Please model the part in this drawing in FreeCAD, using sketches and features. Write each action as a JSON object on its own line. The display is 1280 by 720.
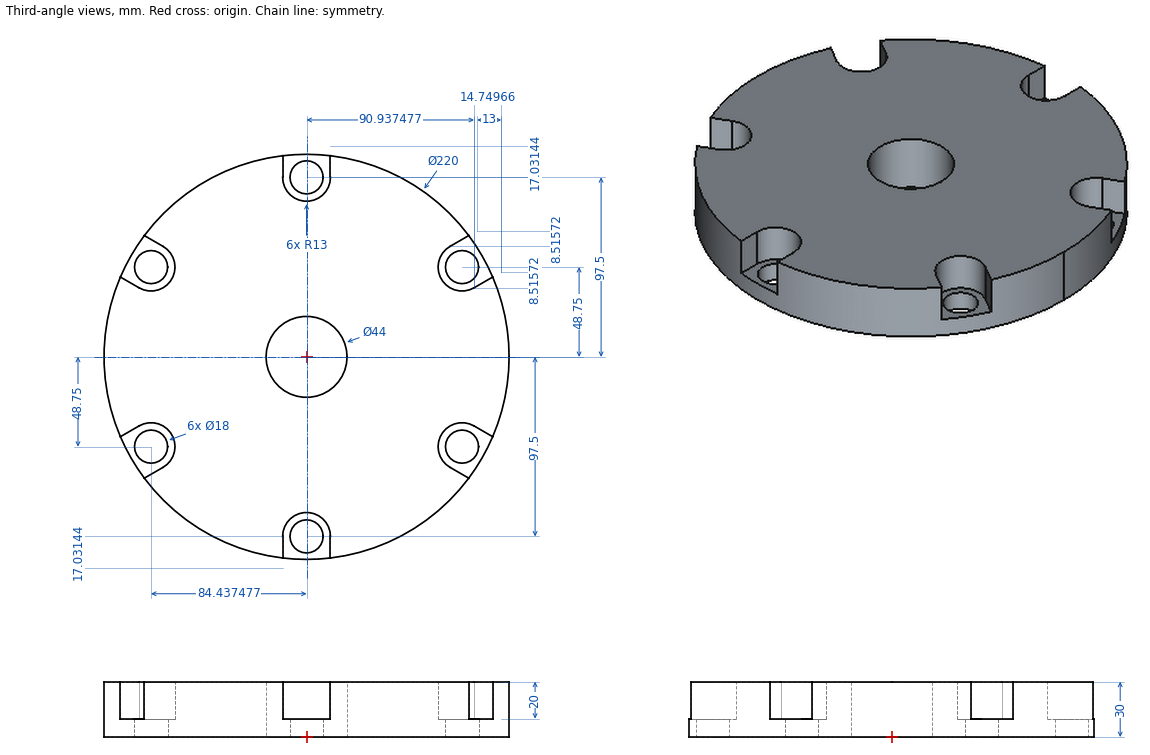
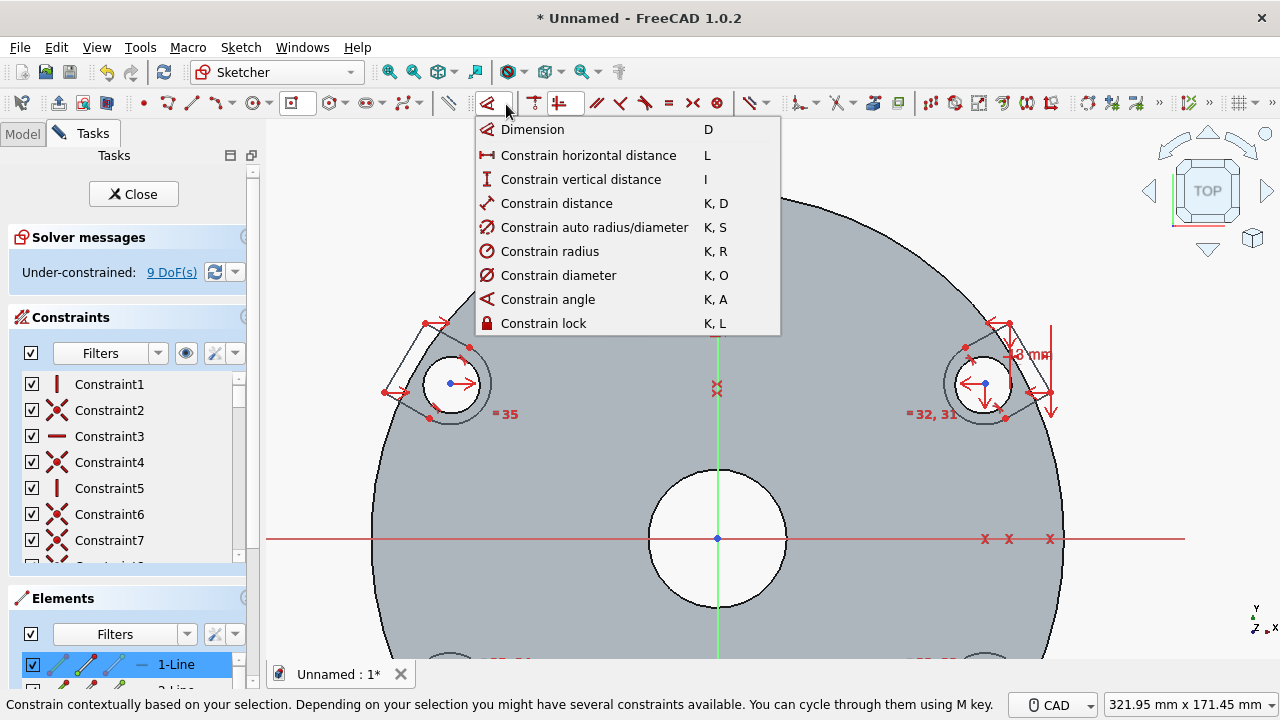
{"action": "left_click", "coordinate": [628, 179]}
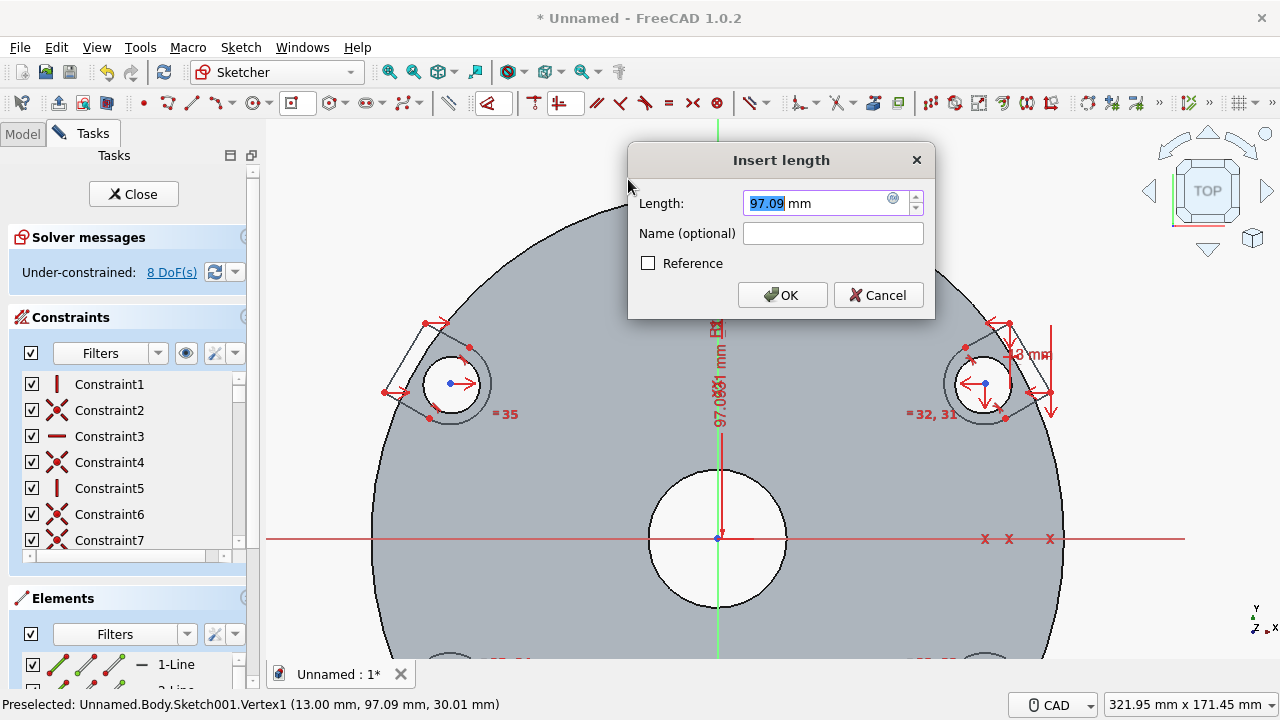
{"action": "type", "text": "97.5"}
{"action": "key", "text": "Return"}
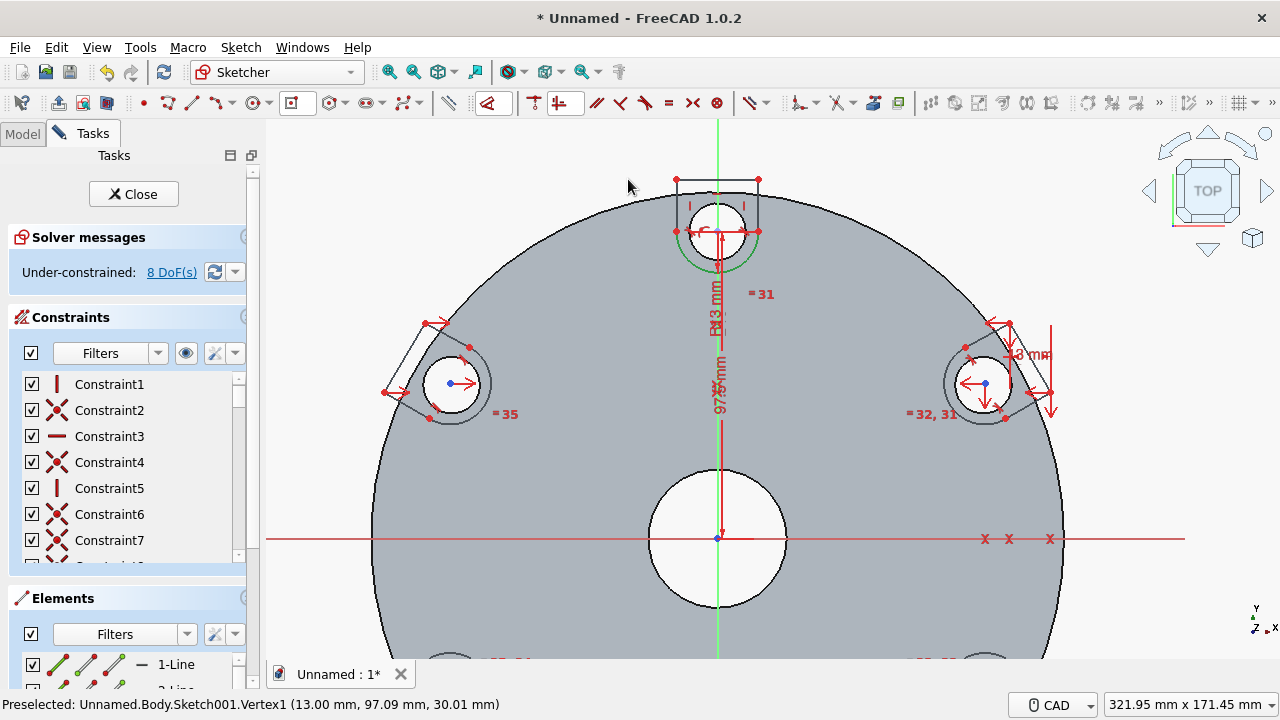
{"action": "scroll", "coordinate": [694, 267], "scroll_direction": "down", "scroll_amount": 4}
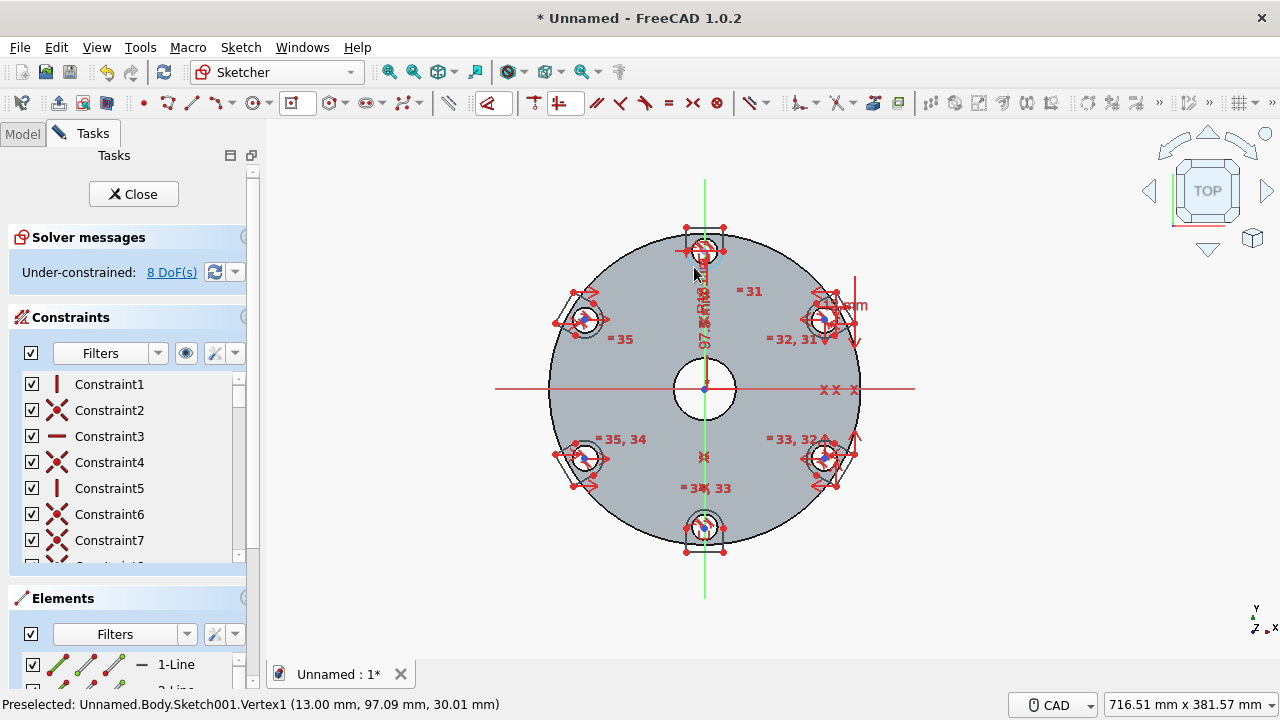
{"action": "left_click", "coordinate": [686, 528]}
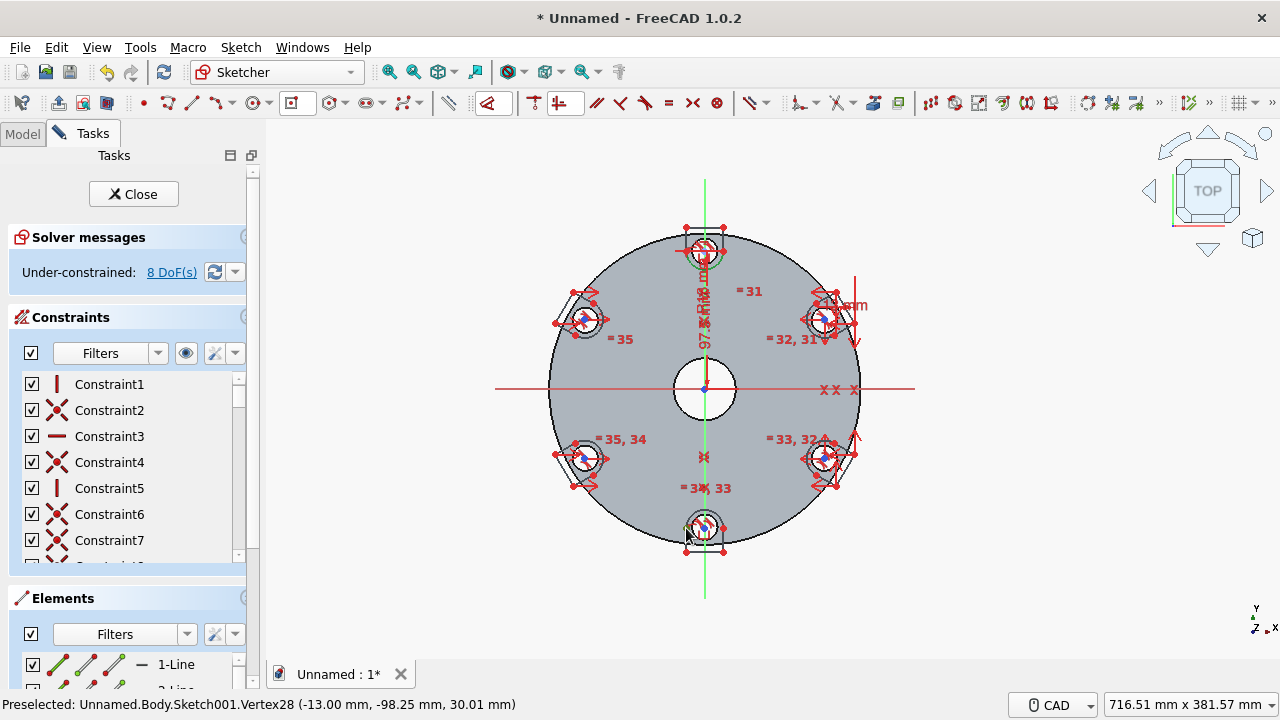
{"action": "left_click", "coordinate": [506, 104]}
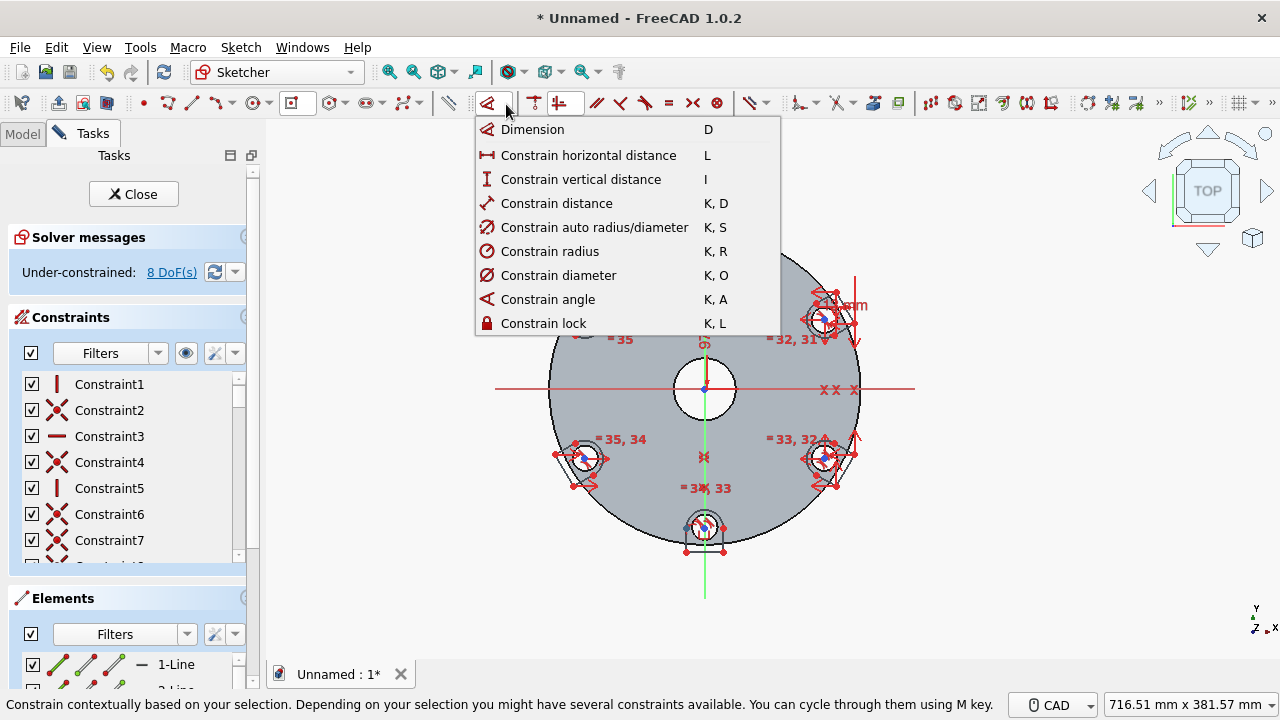
{"action": "left_click", "coordinate": [628, 179]}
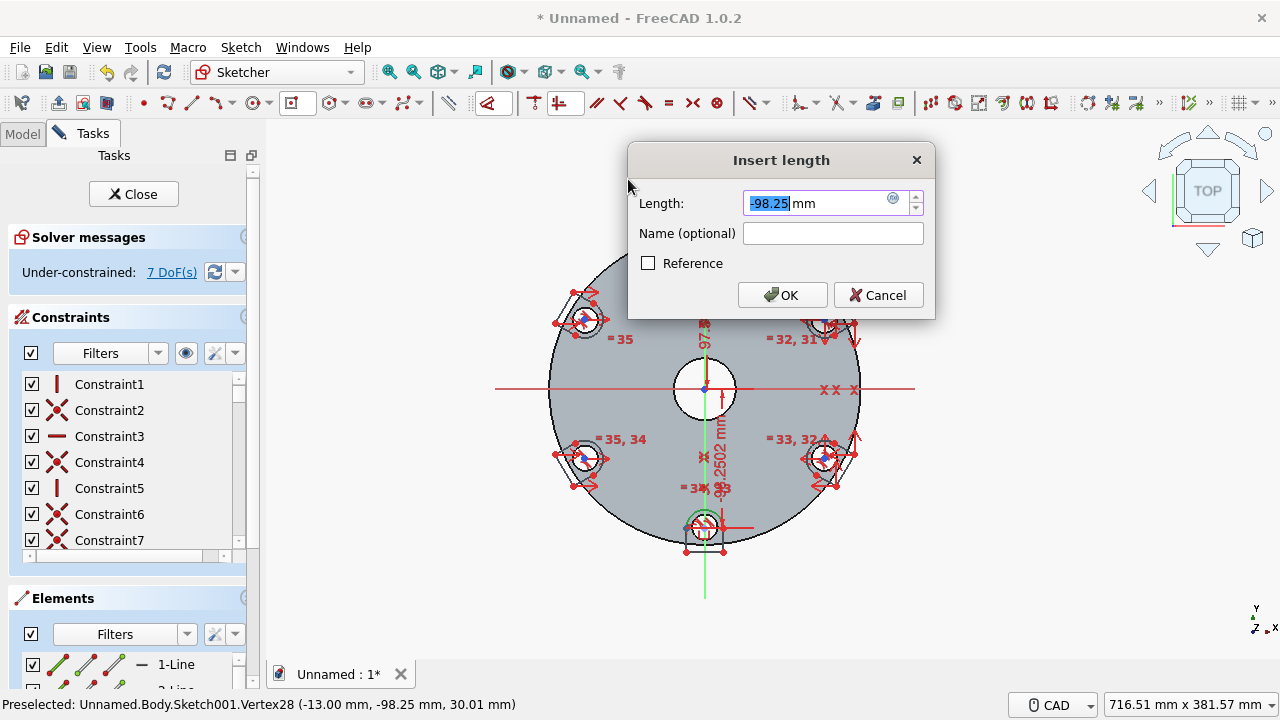
{"action": "type", "text": "-97.5"}
{"action": "key", "text": "Return"}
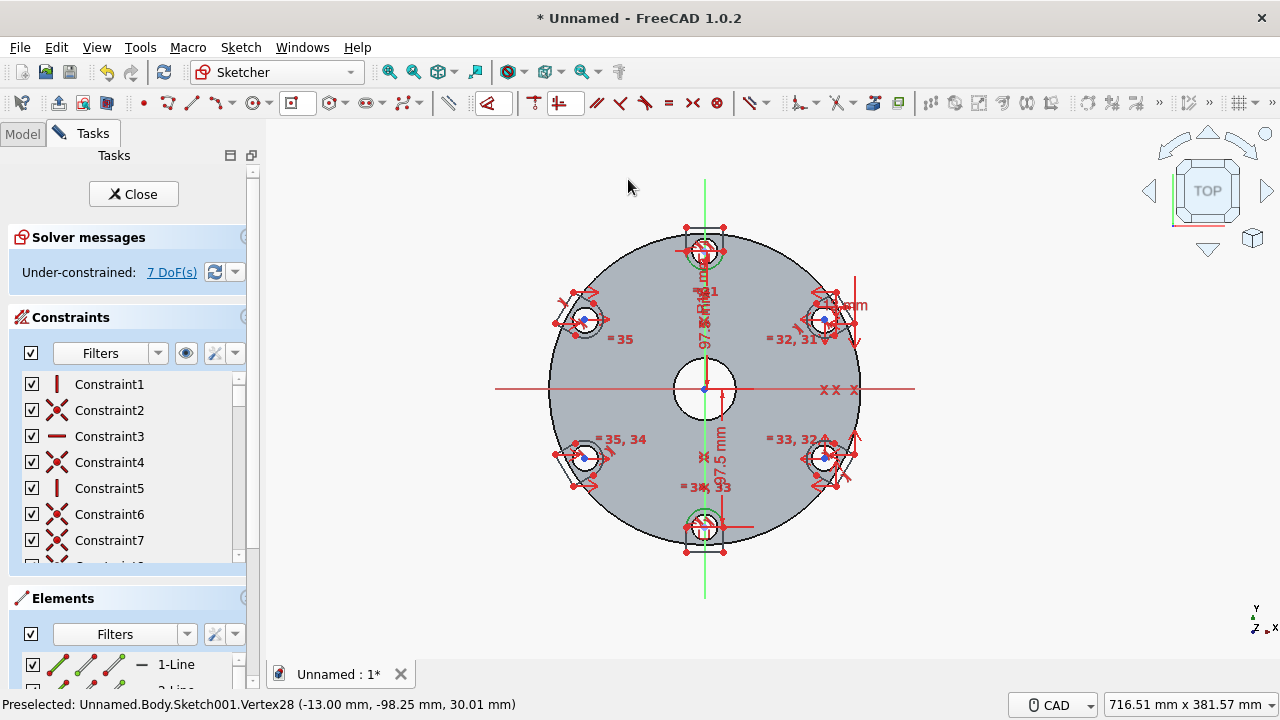
{"action": "left_click", "coordinate": [825, 320]}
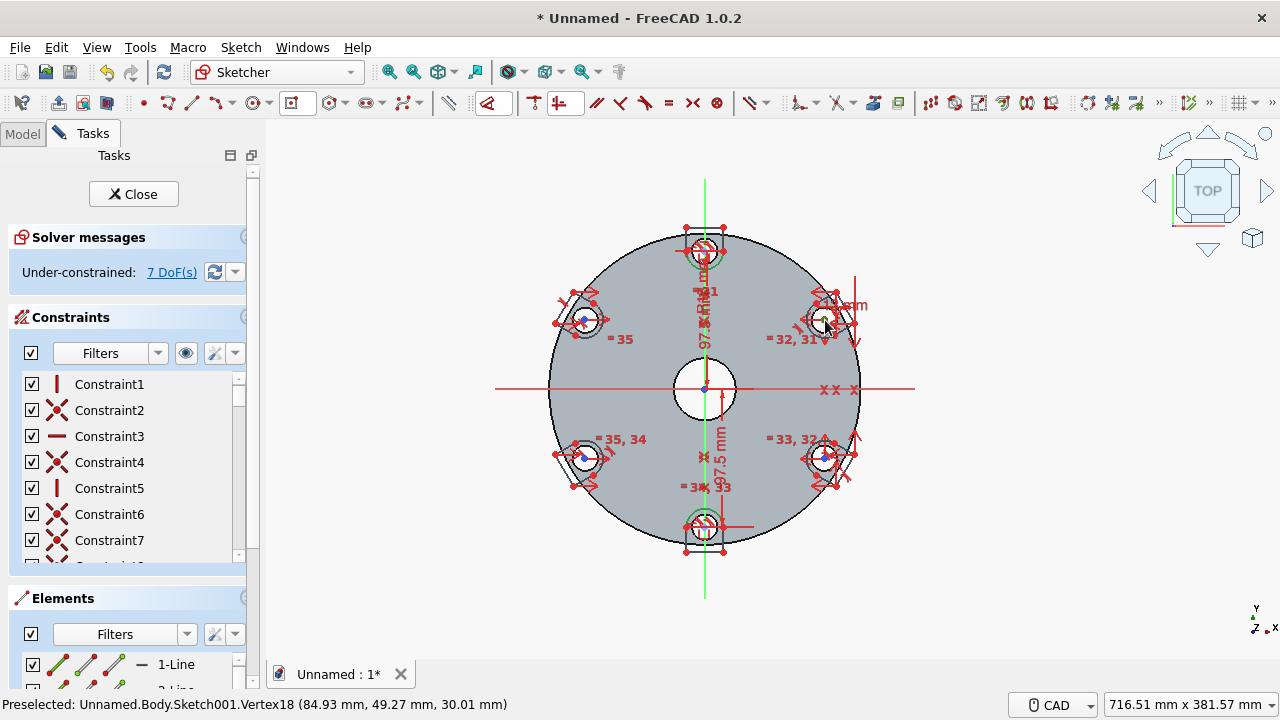
{"action": "key", "text": "i"}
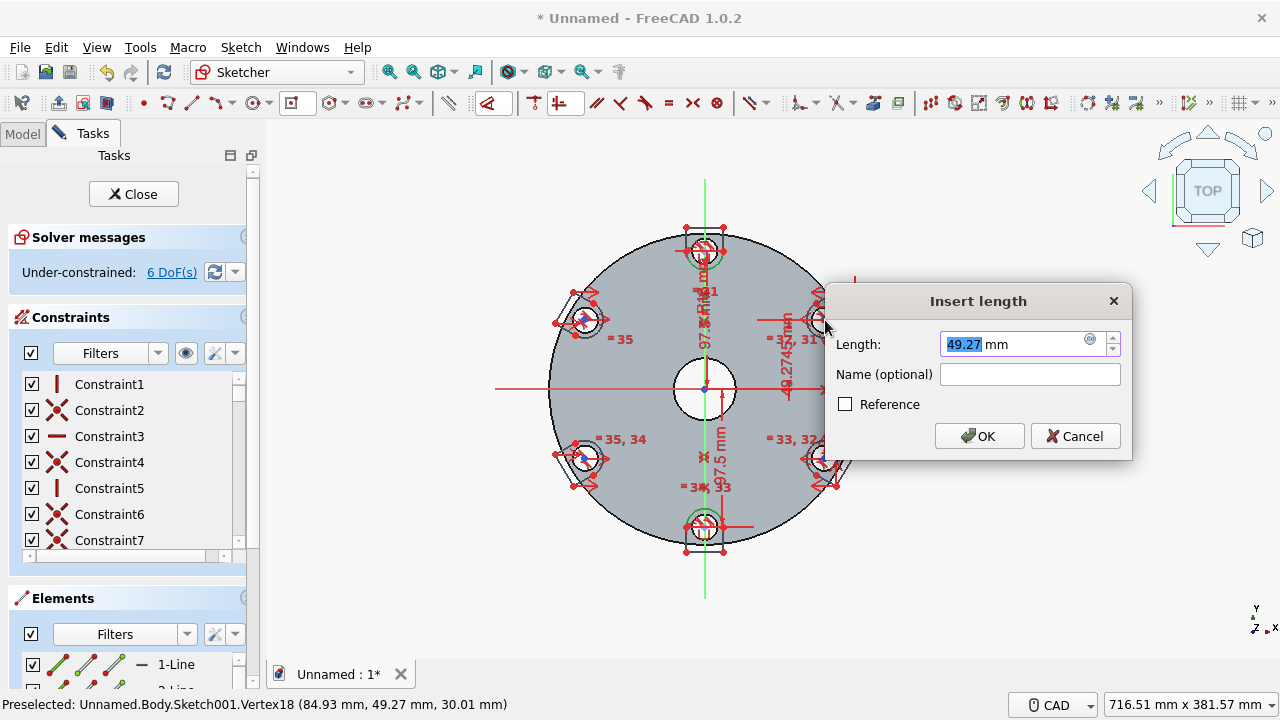
{"action": "type", "text": "48.75"}
{"action": "key", "text": "Return"}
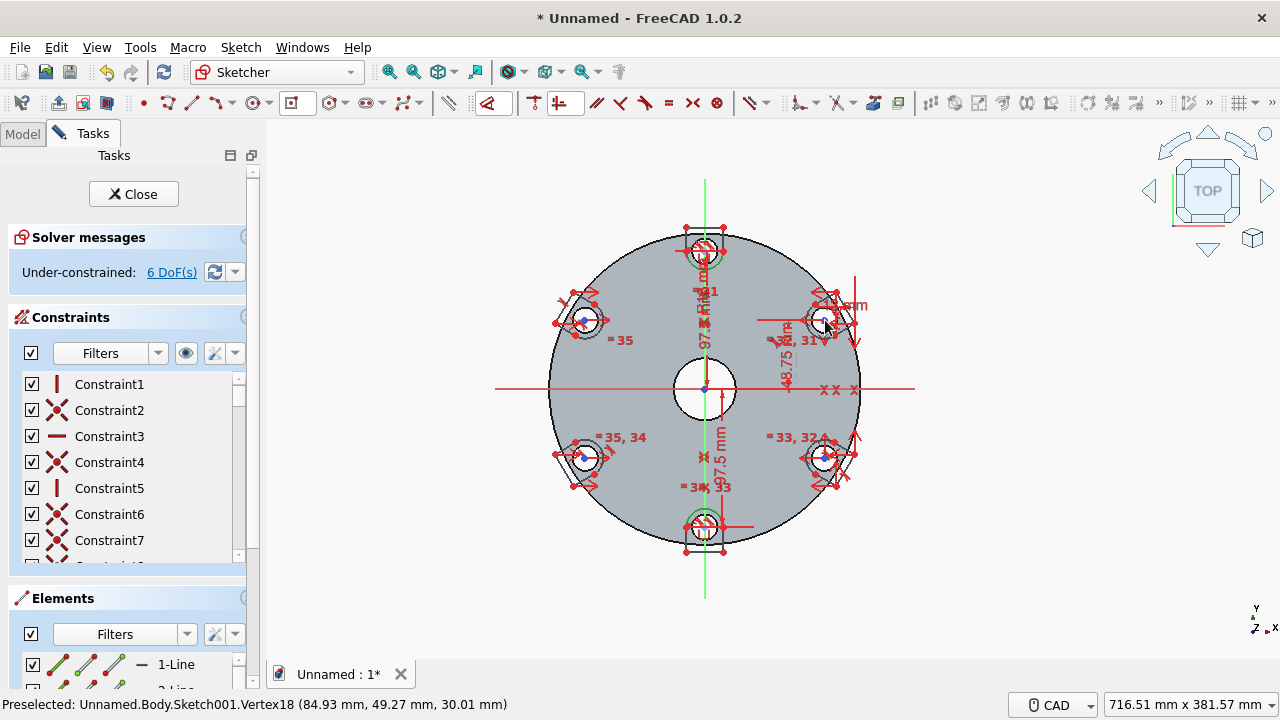
{"action": "scroll", "coordinate": [723, 242], "scroll_direction": "up", "scroll_amount": 3}